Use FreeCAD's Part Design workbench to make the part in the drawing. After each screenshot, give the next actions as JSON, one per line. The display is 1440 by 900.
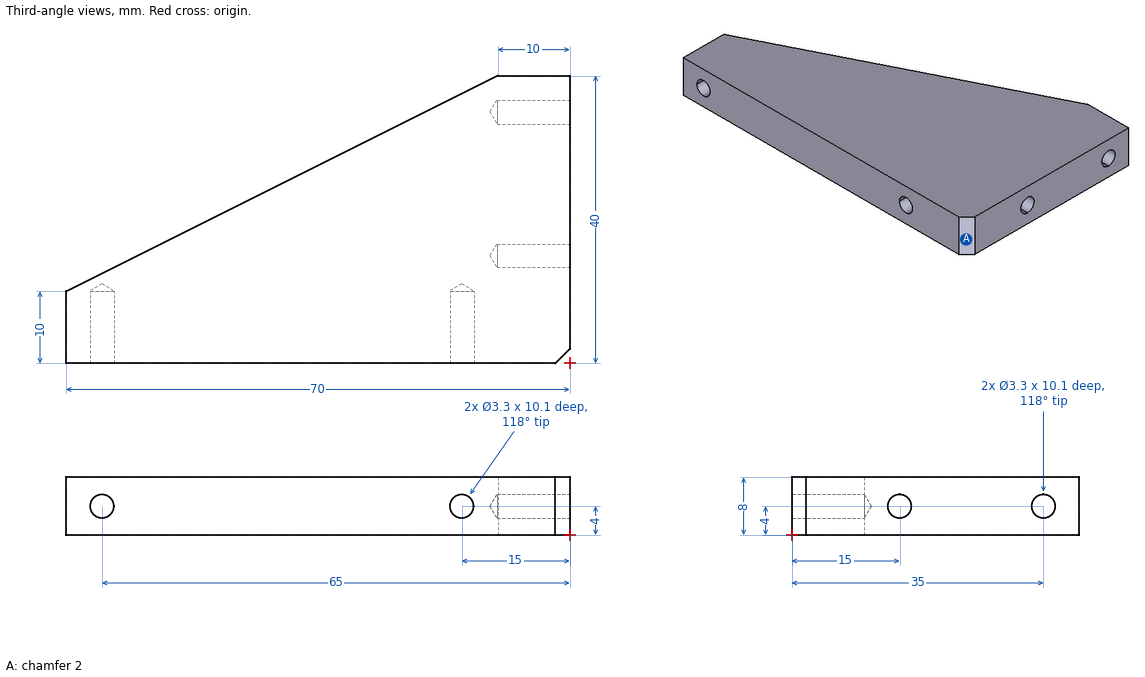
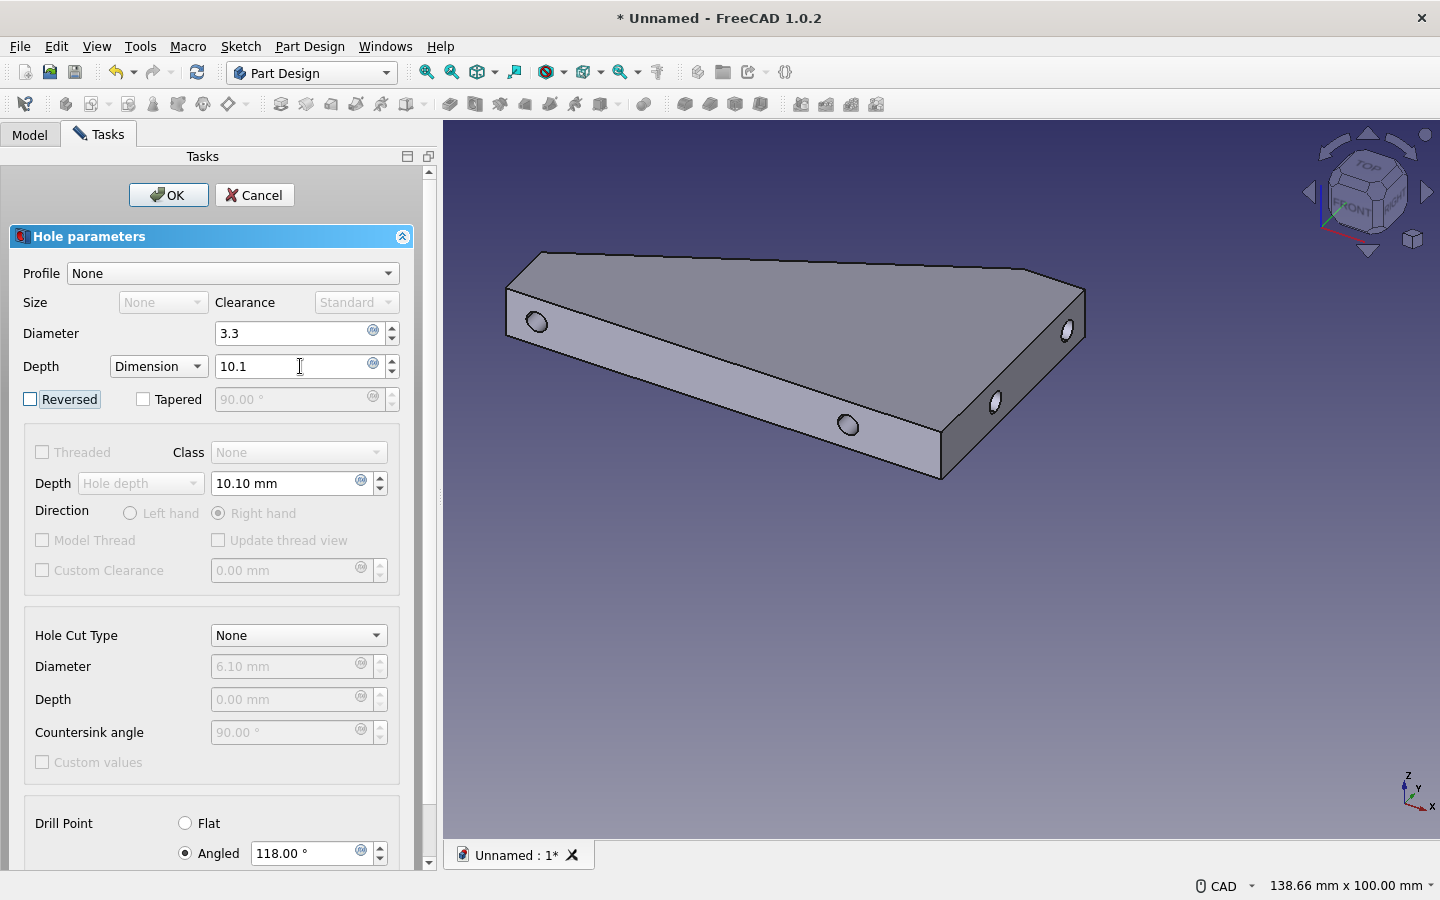
{"action": "left_click", "coordinate": [169, 195]}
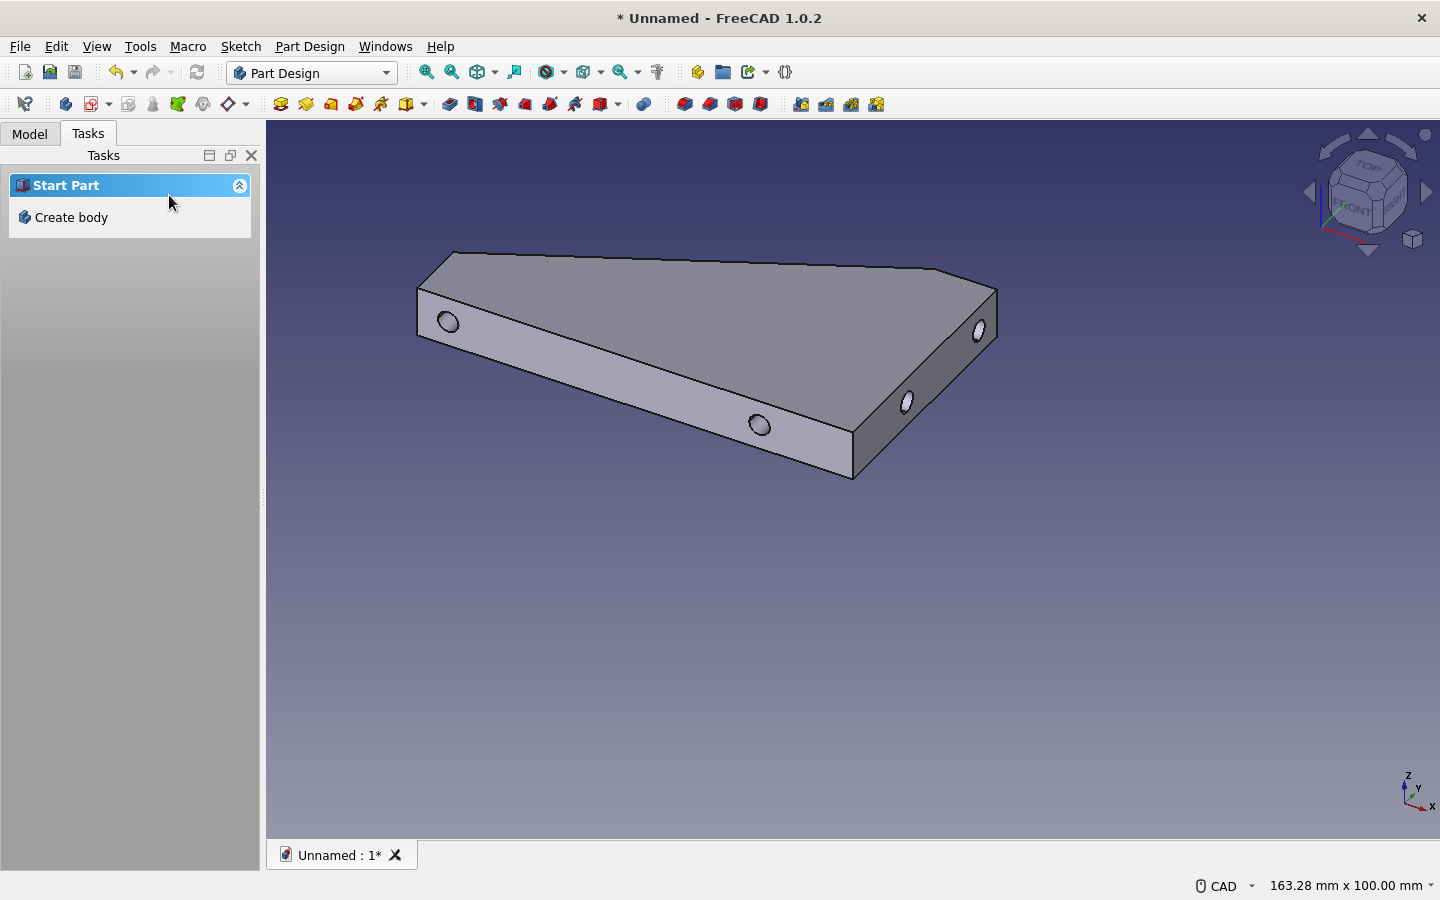
{"action": "left_click", "coordinate": [853, 455]}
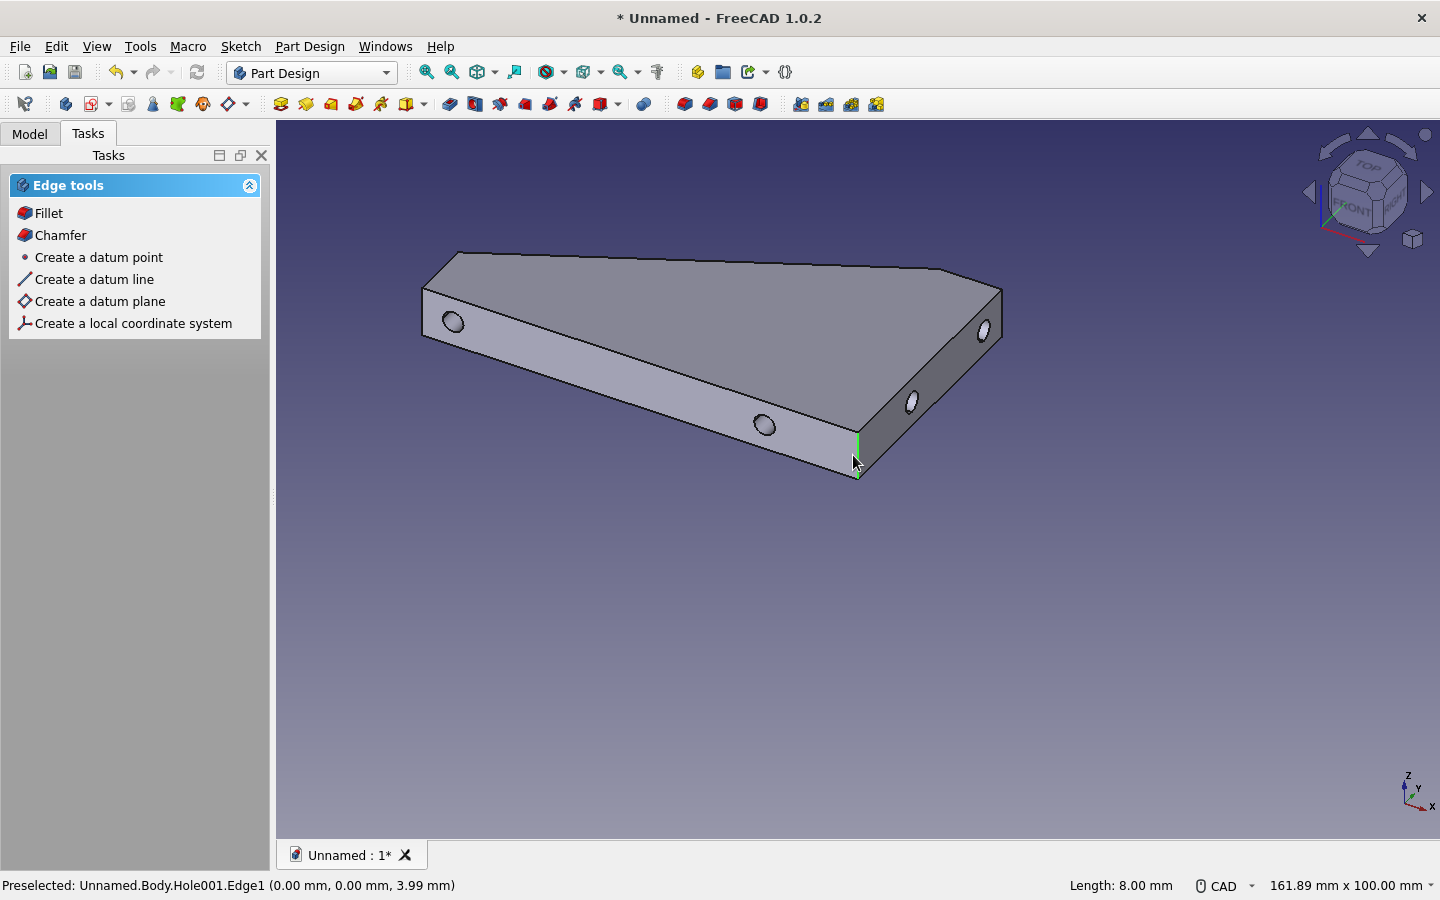
{"action": "left_click", "coordinate": [710, 104]}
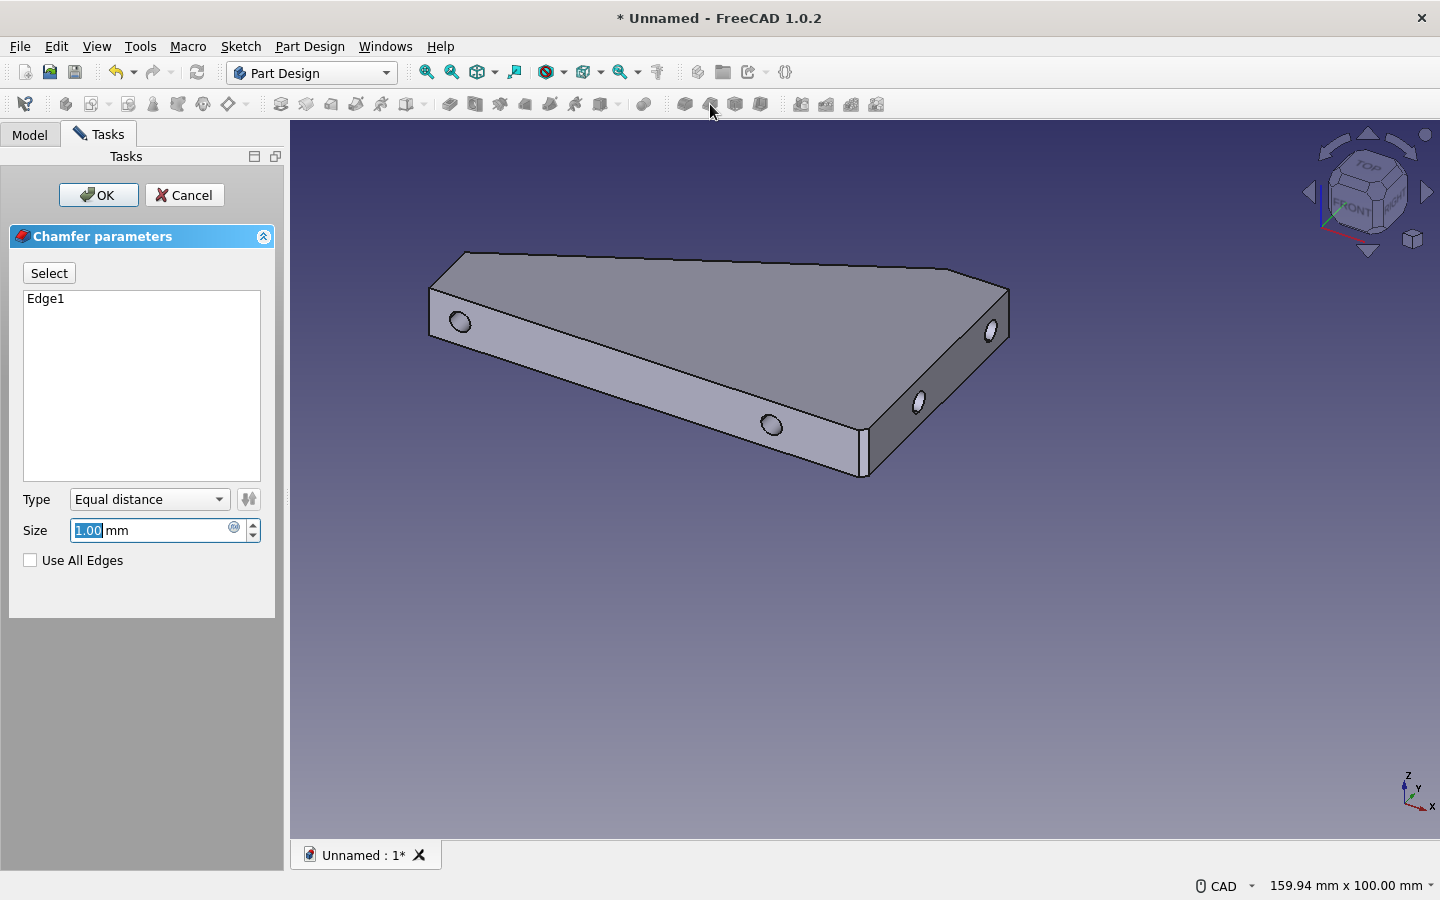
{"action": "type", "text": "2"}
{"action": "key", "text": "Tab"}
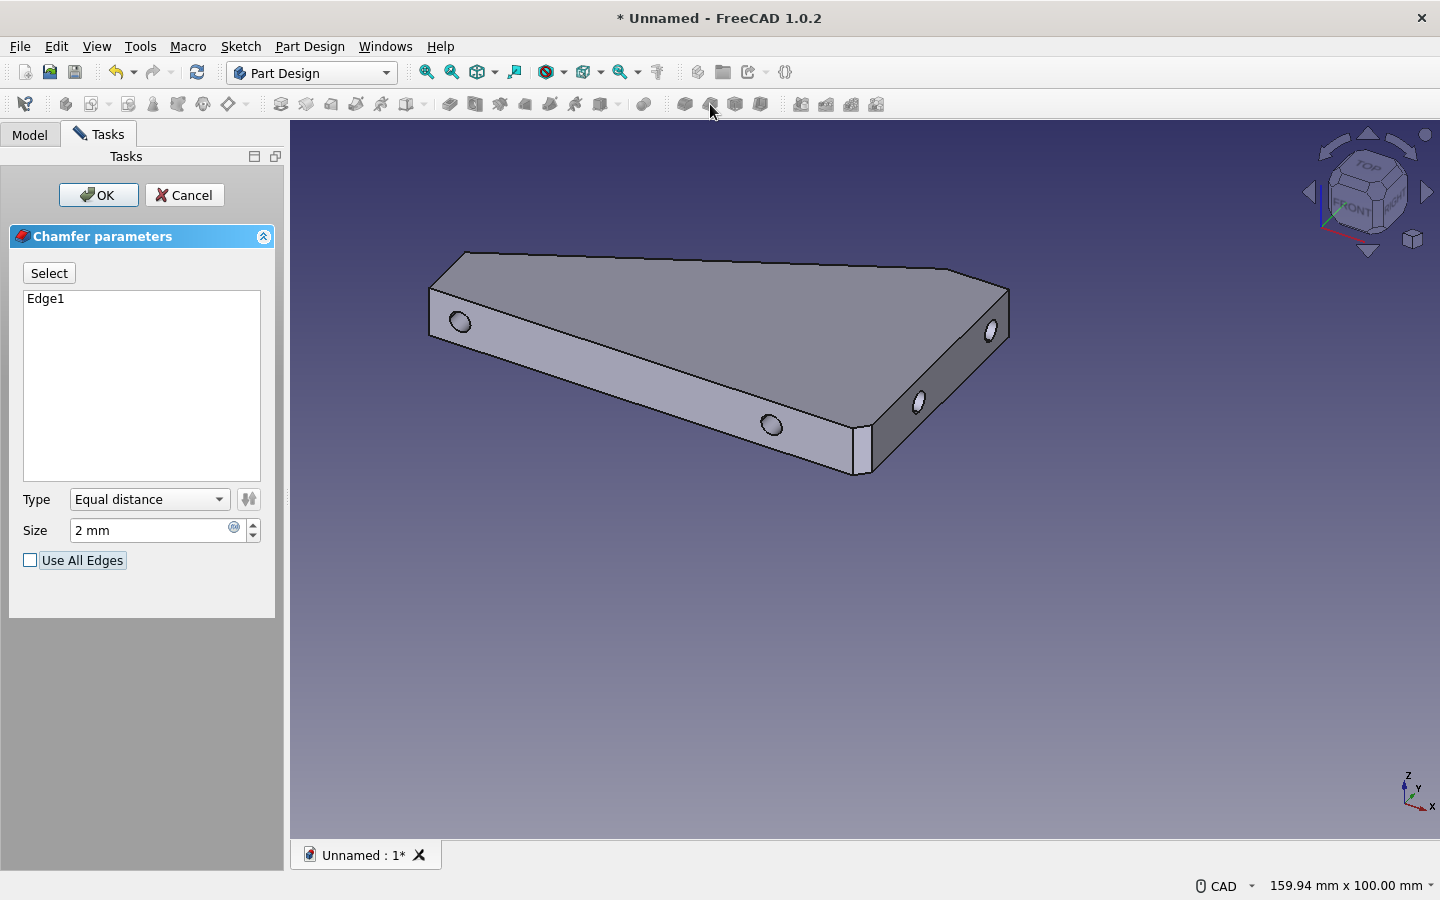
{"action": "left_click", "coordinate": [99, 195]}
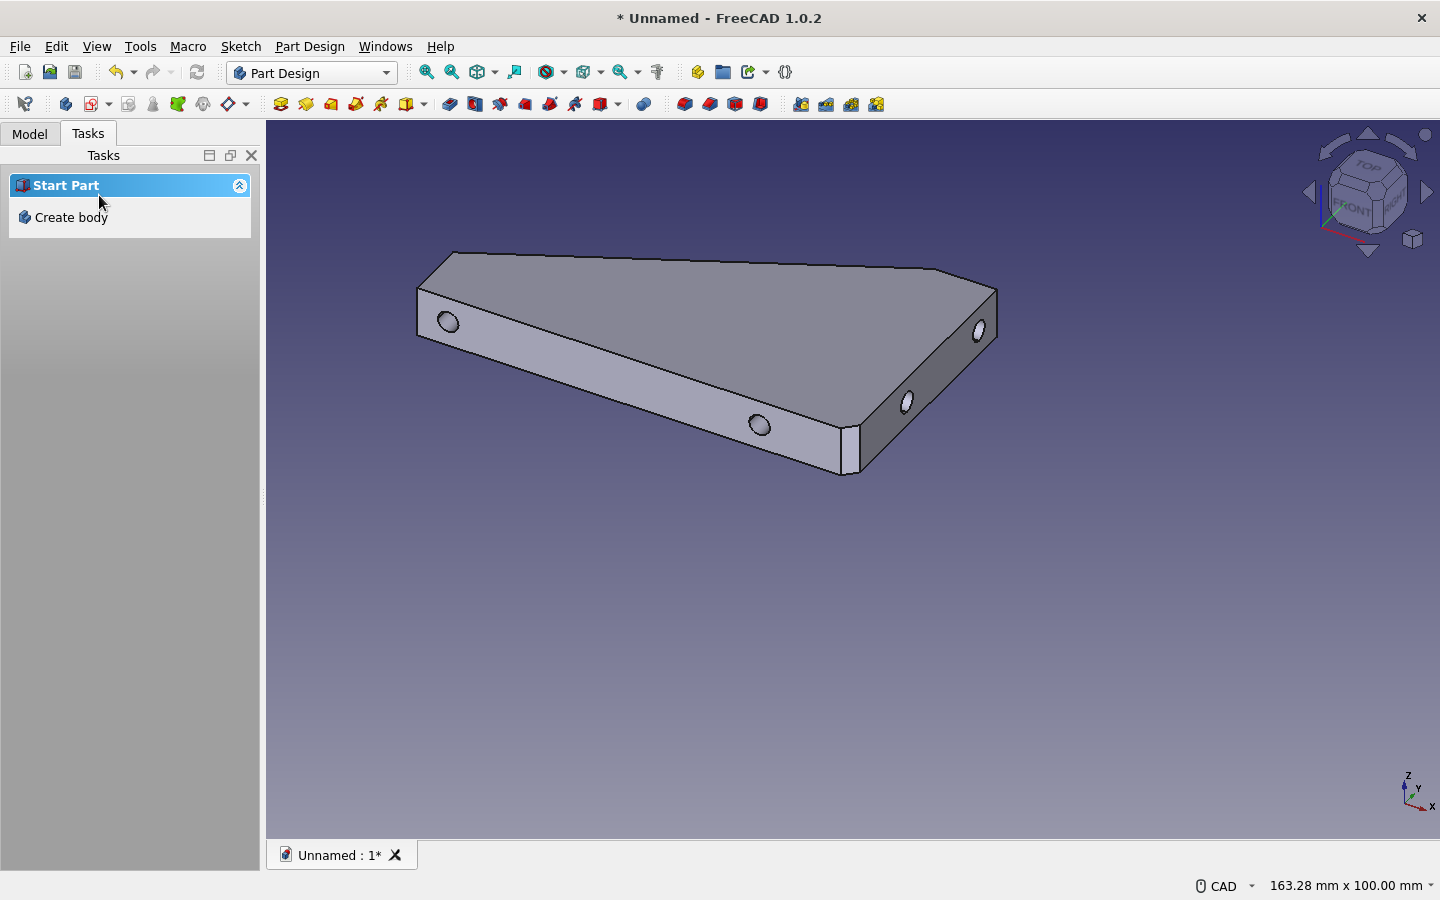
{"action": "key", "text": "0"}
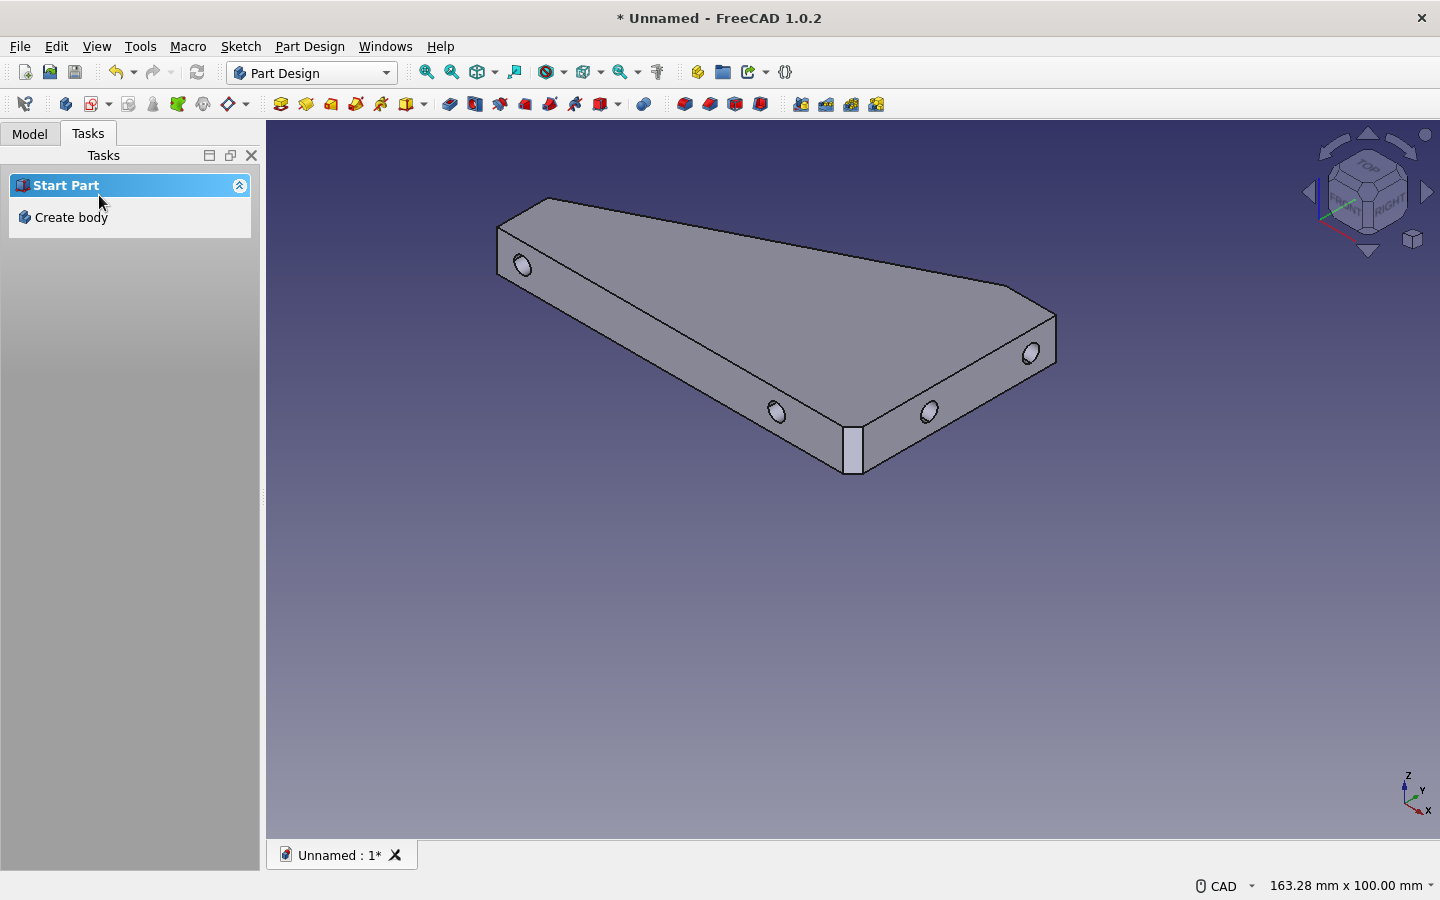
{"action": "left_click", "coordinate": [427, 72]}